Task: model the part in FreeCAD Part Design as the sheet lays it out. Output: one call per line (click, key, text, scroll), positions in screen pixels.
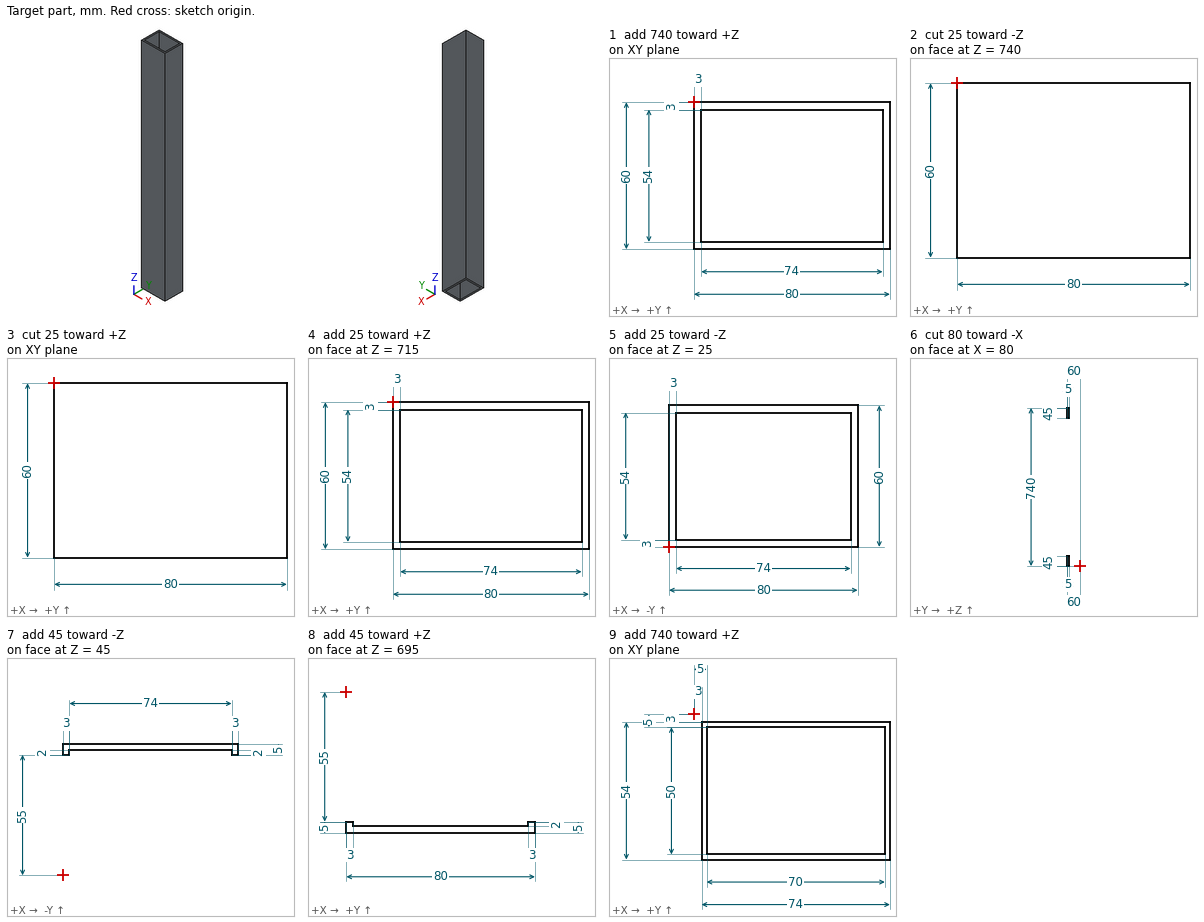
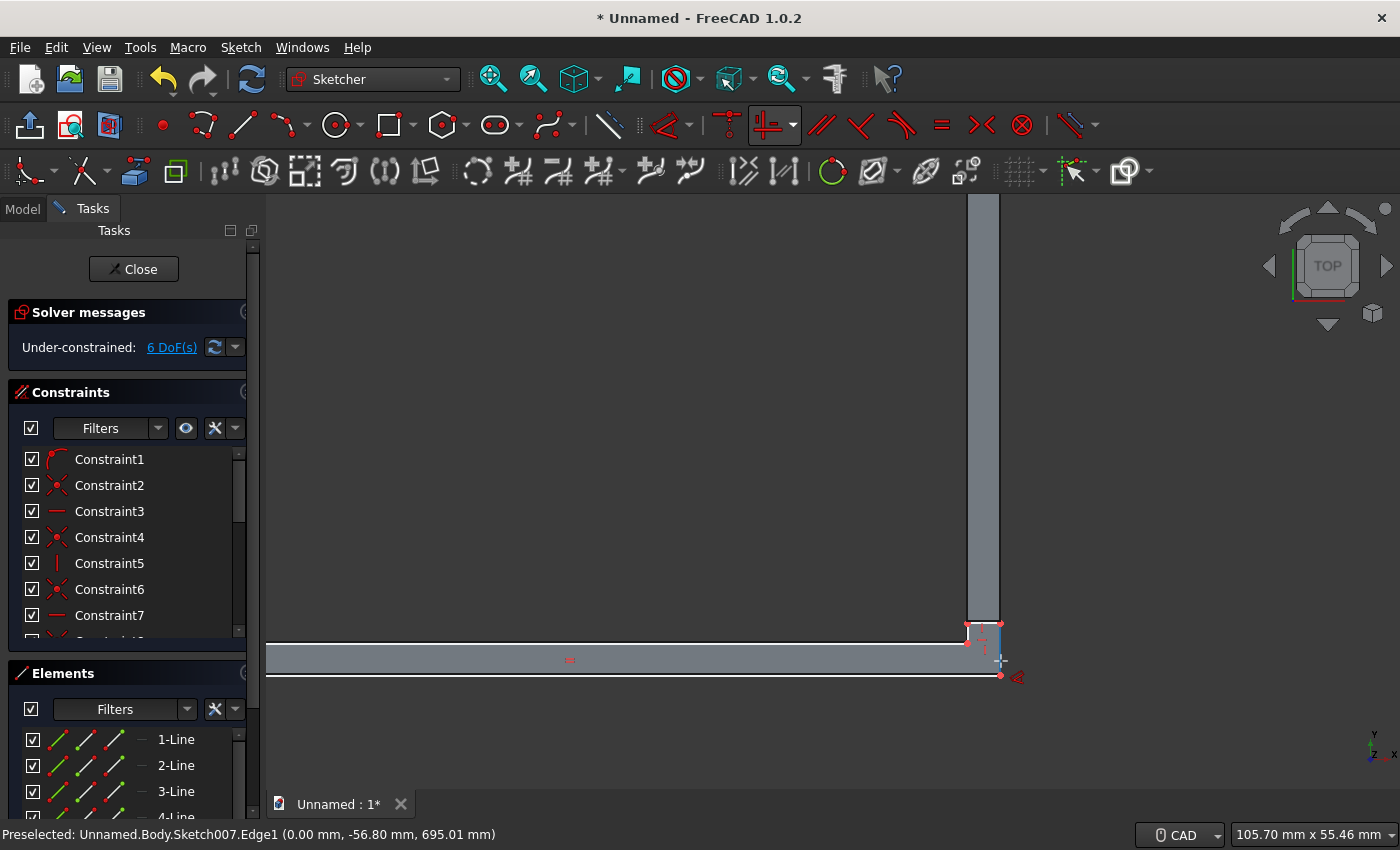
click(1000, 660)
click(1034, 649)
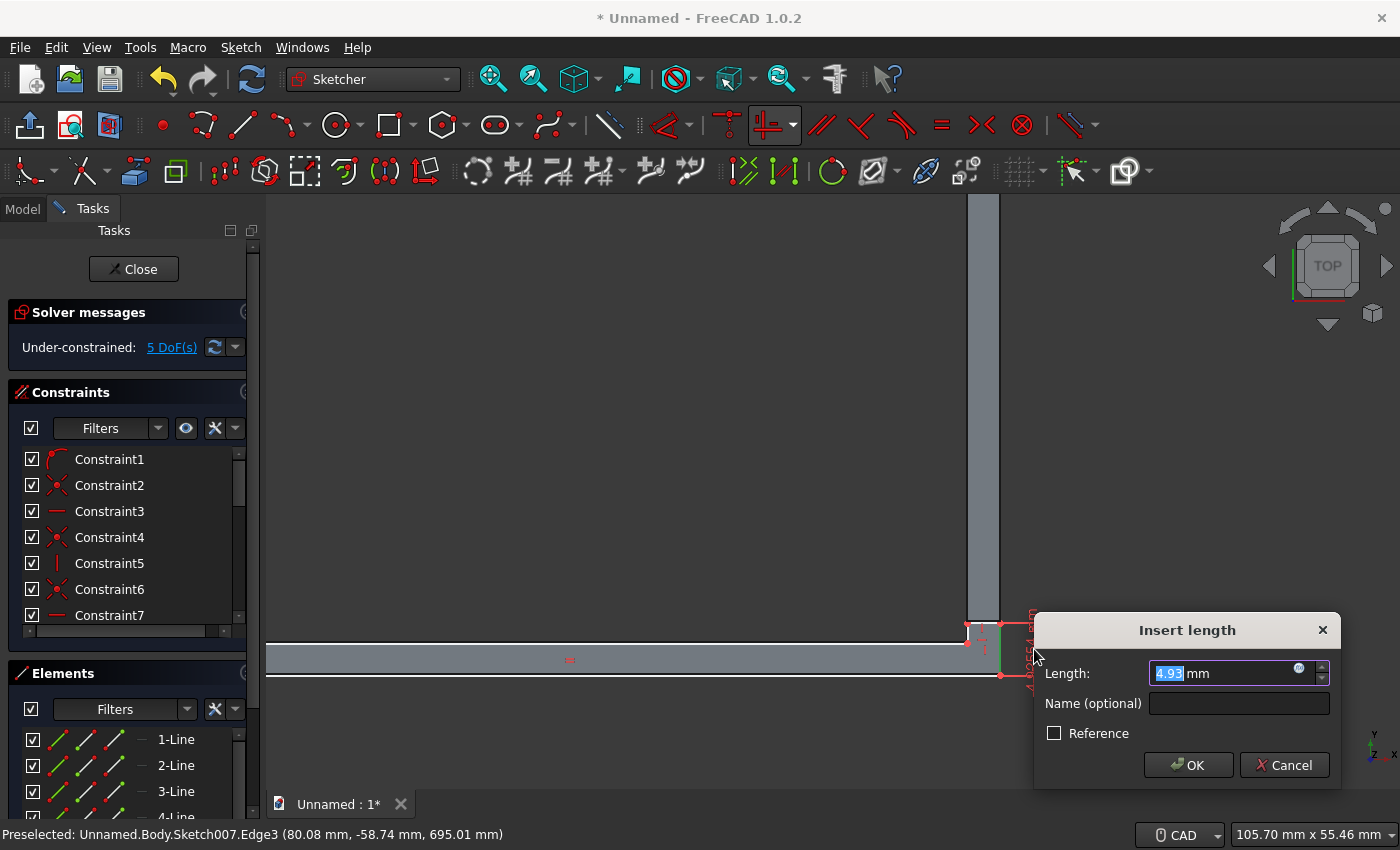
text(5)
key(Return)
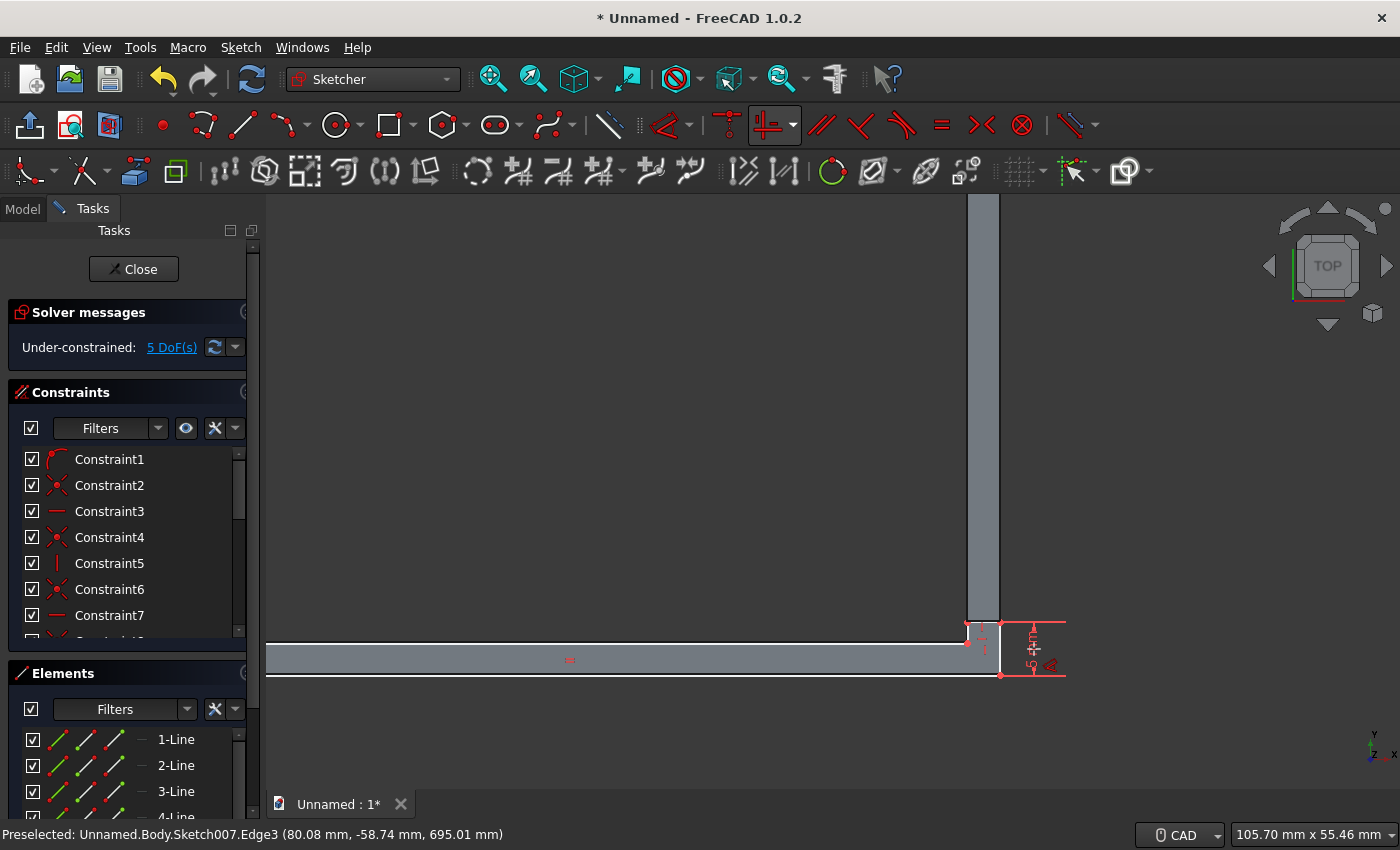
scroll(990, 622, up, 2)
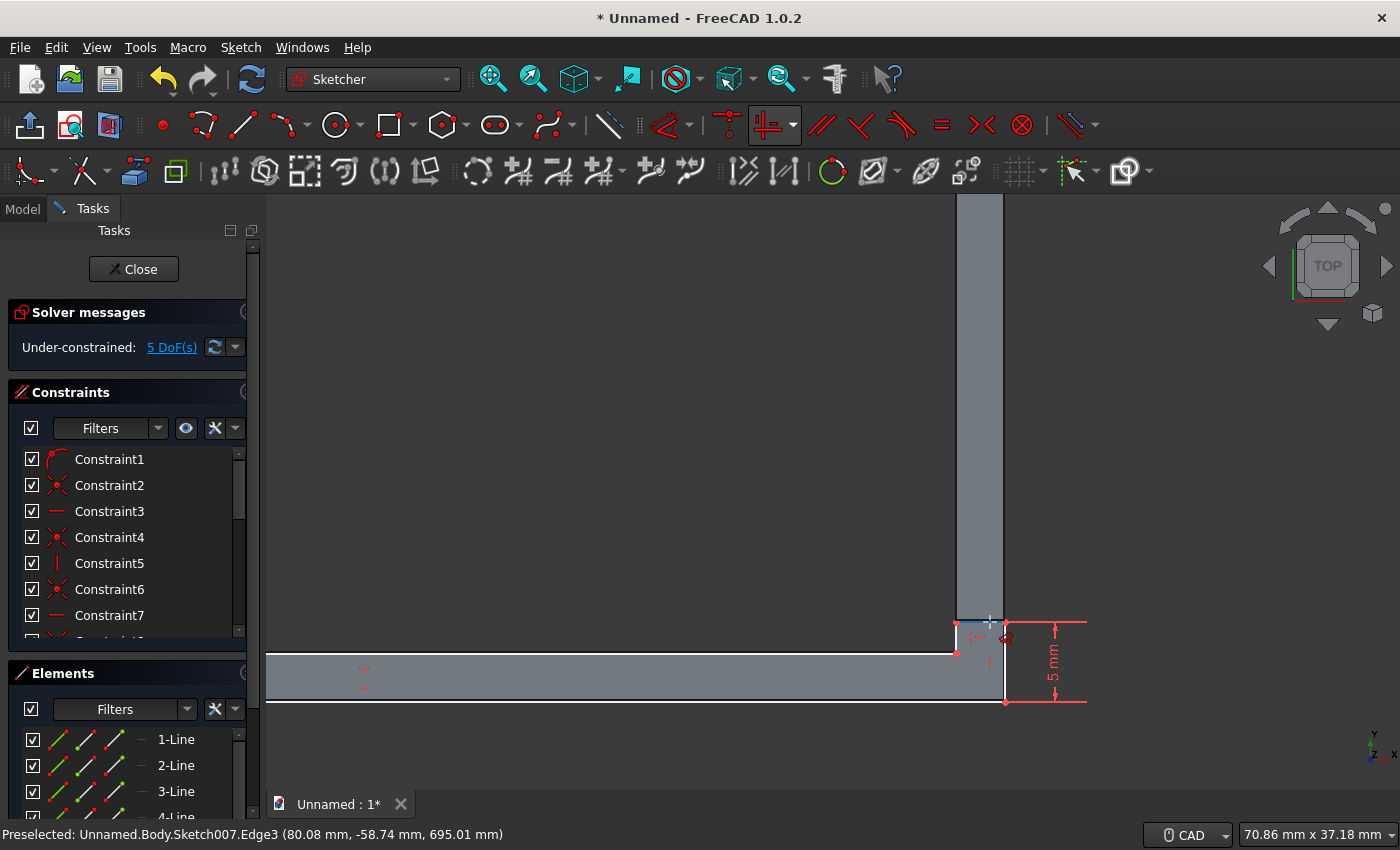
click(990, 622)
click(981, 656)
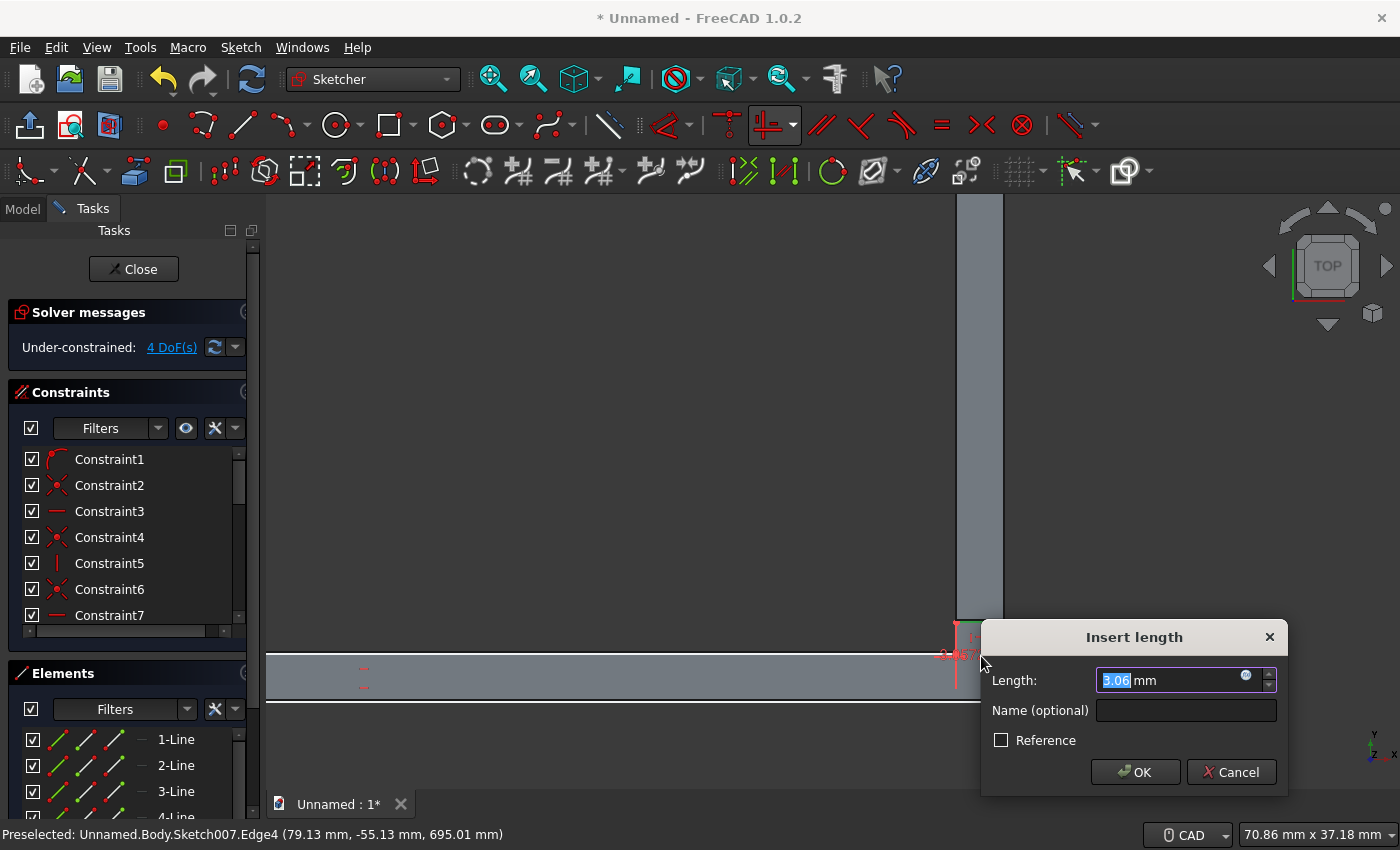
text(3)
key(Return)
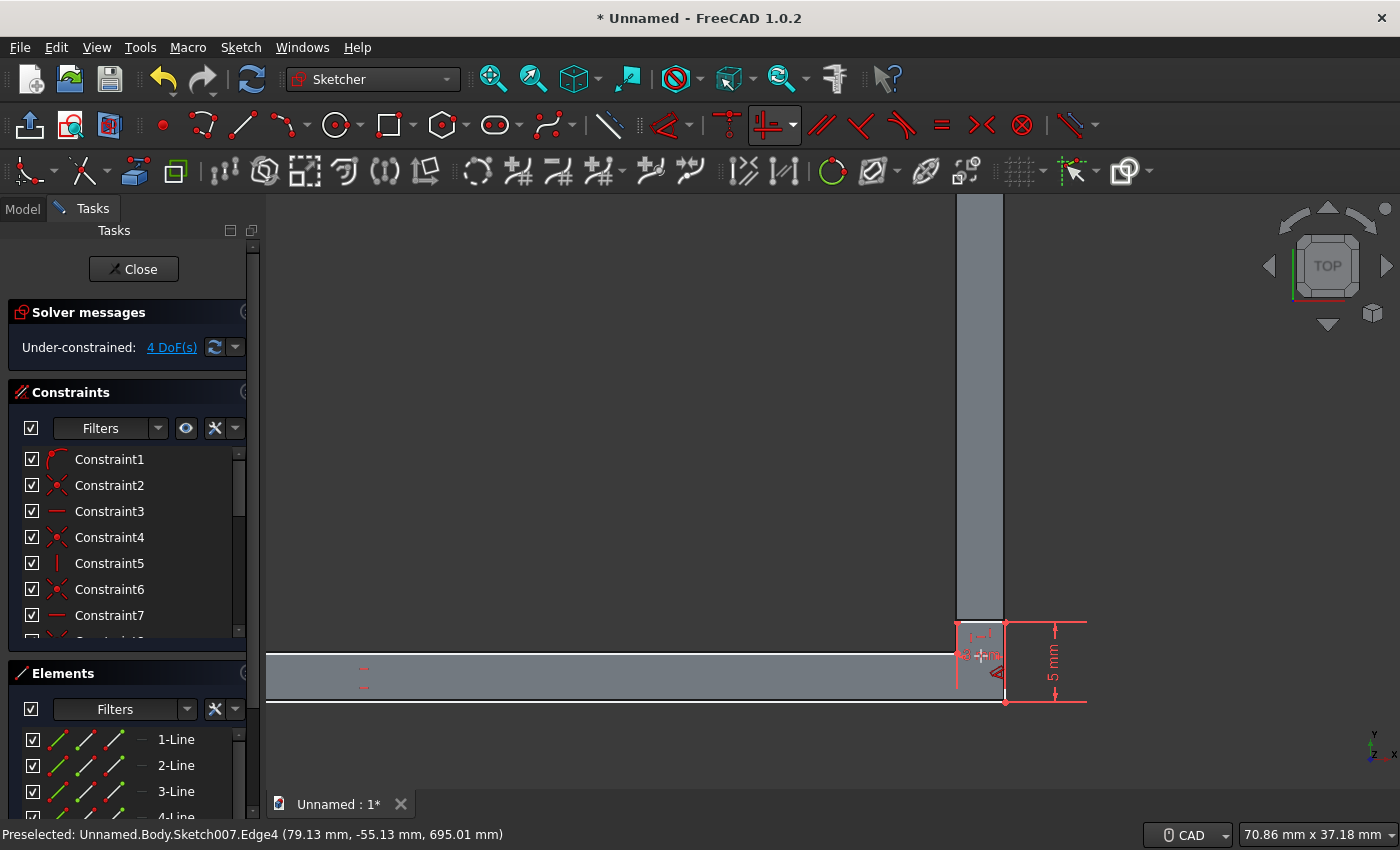
scroll(957, 632, up, 2)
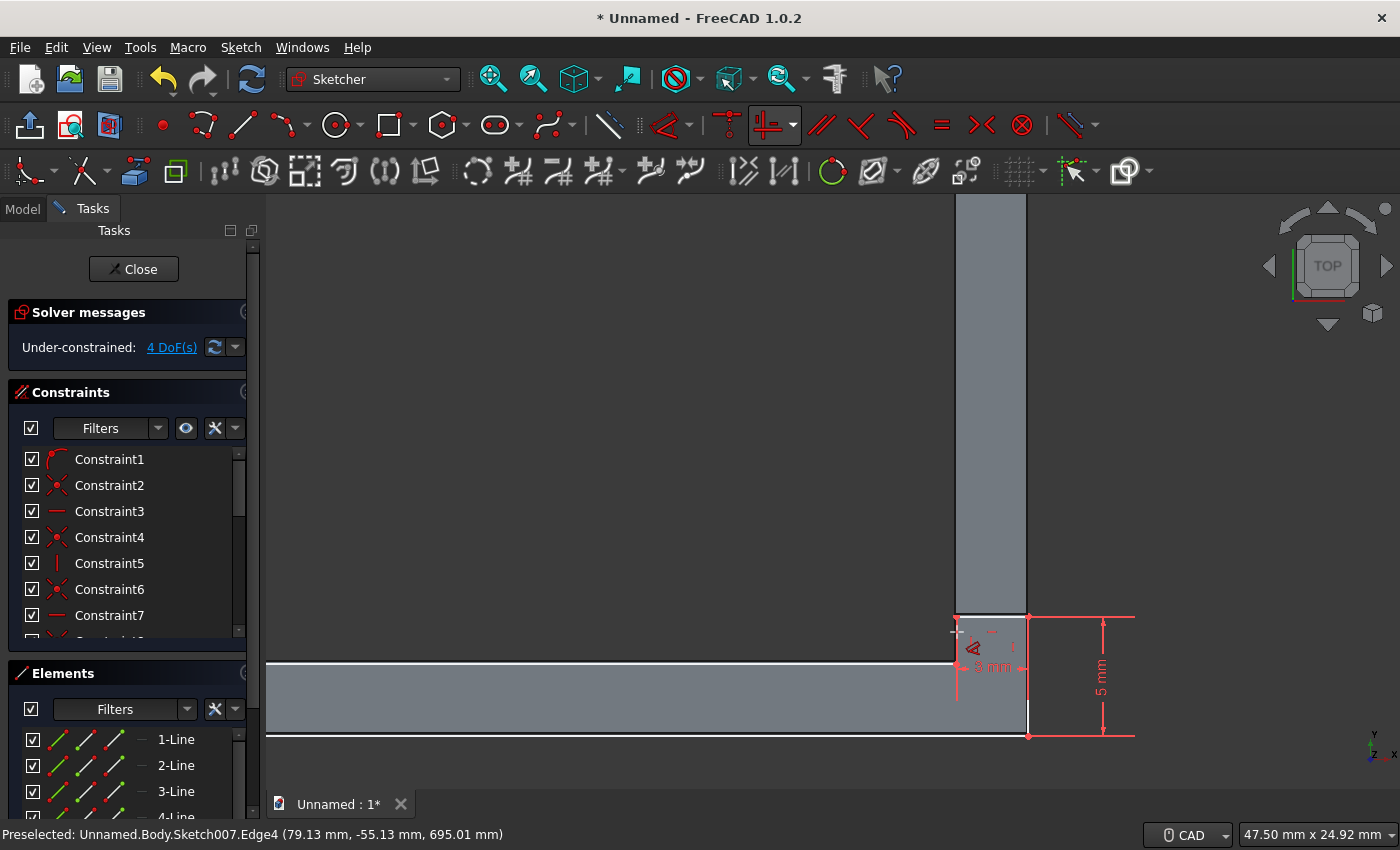
click(957, 631)
click(991, 640)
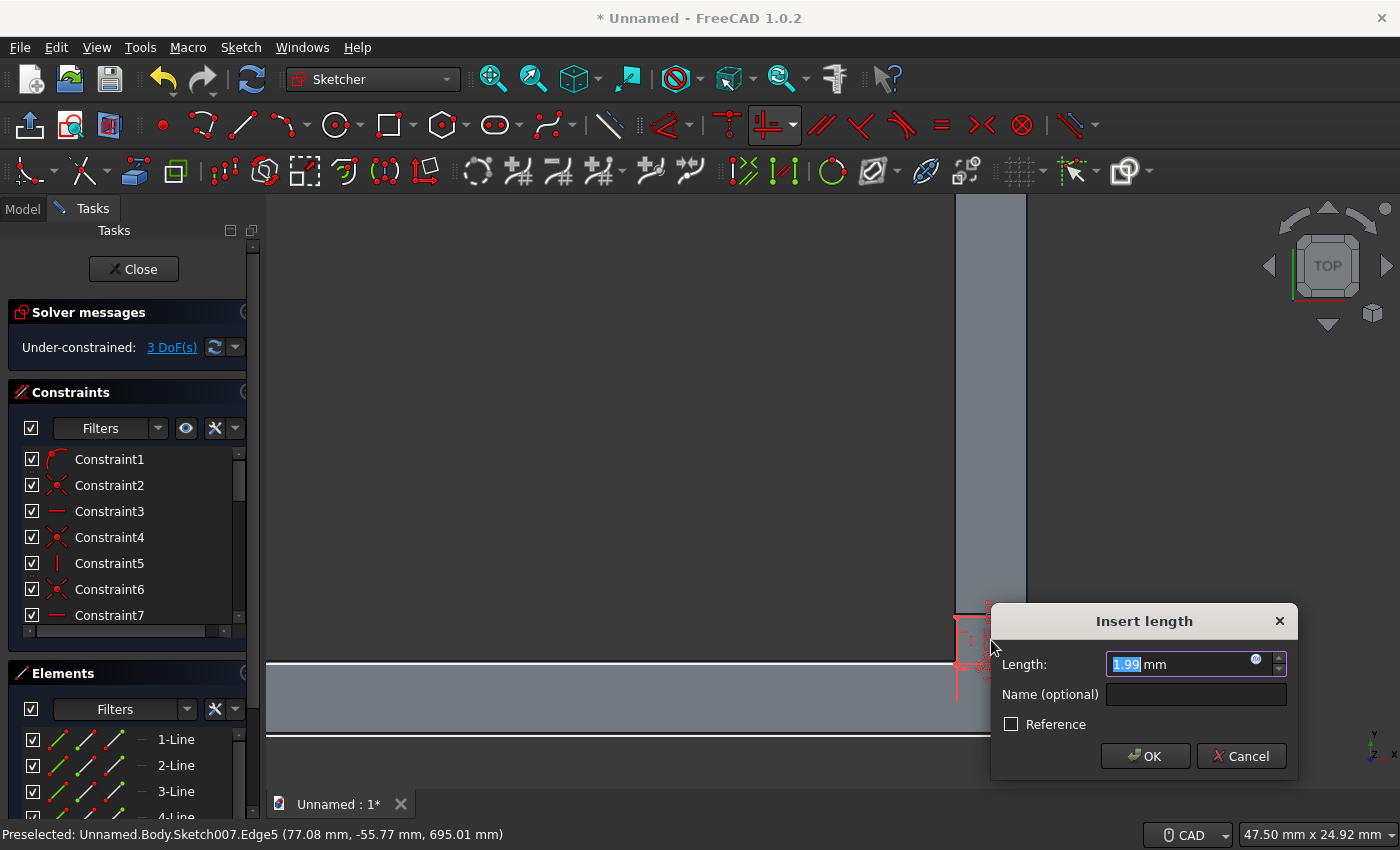
text(2)
key(Return)